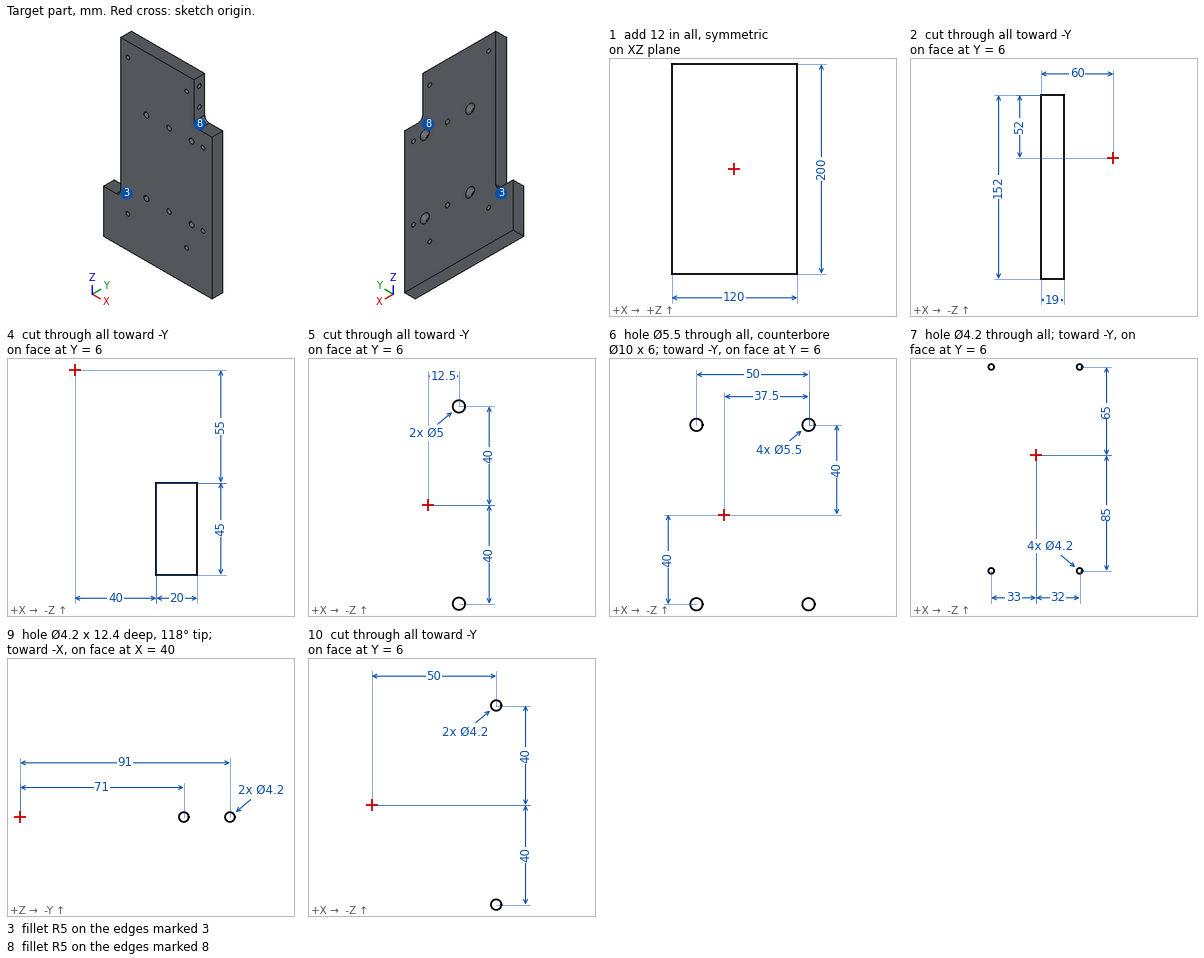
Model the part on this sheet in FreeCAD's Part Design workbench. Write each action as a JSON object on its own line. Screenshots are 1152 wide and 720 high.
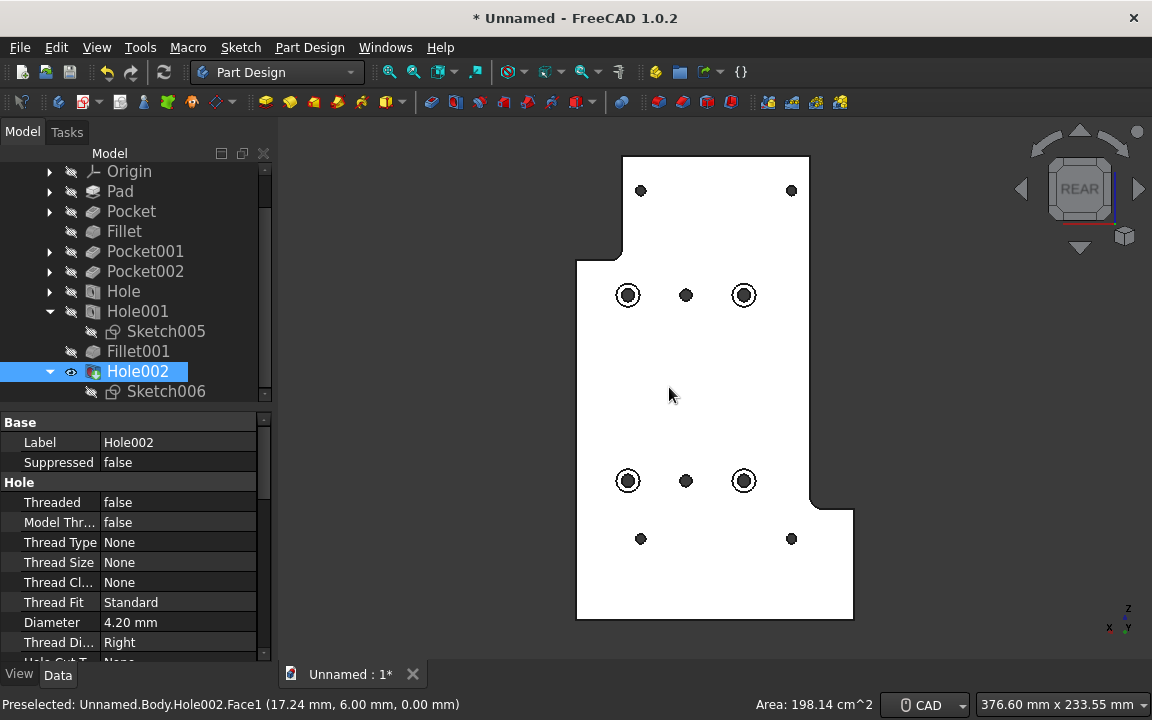
{"action": "left_click", "coordinate": [84, 102]}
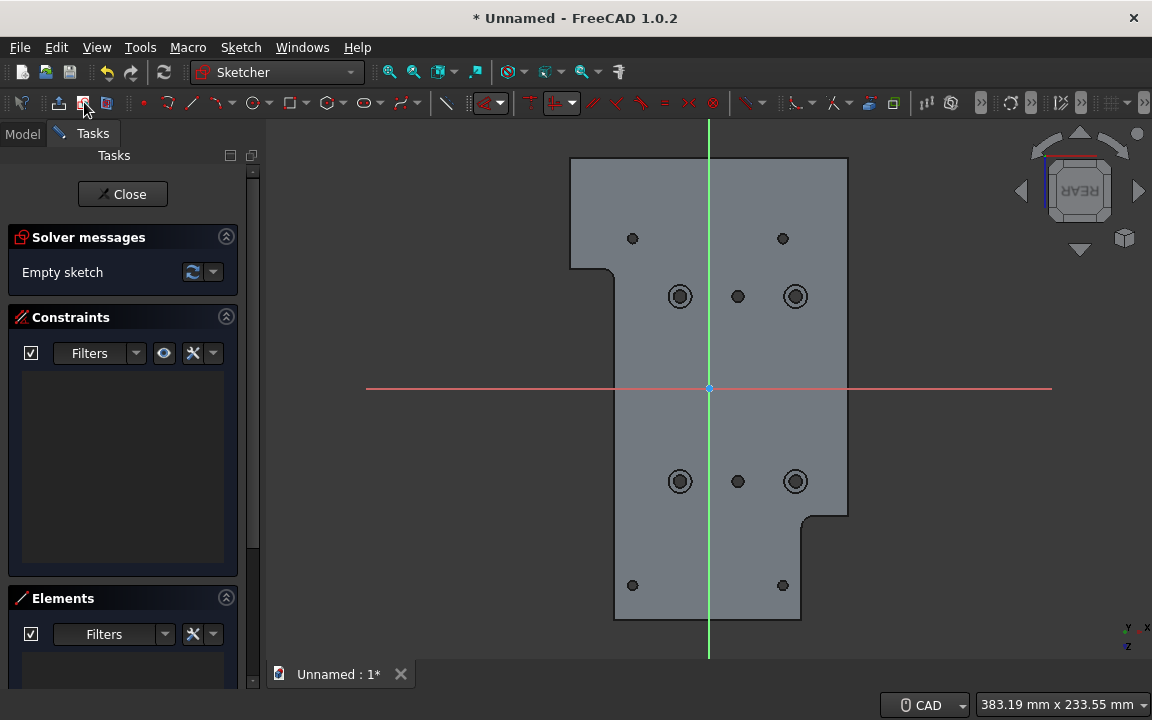
{"action": "scroll", "coordinate": [926, 389], "scroll_direction": "up", "scroll_amount": 3}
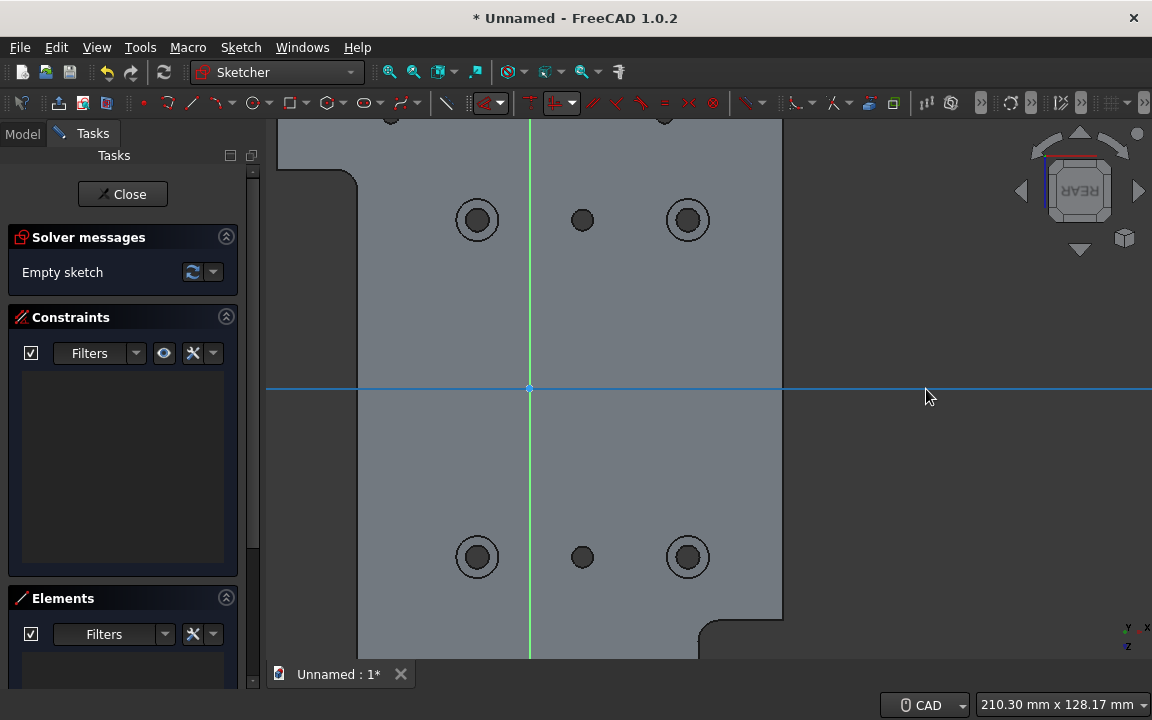
{"action": "left_click", "coordinate": [254, 104]}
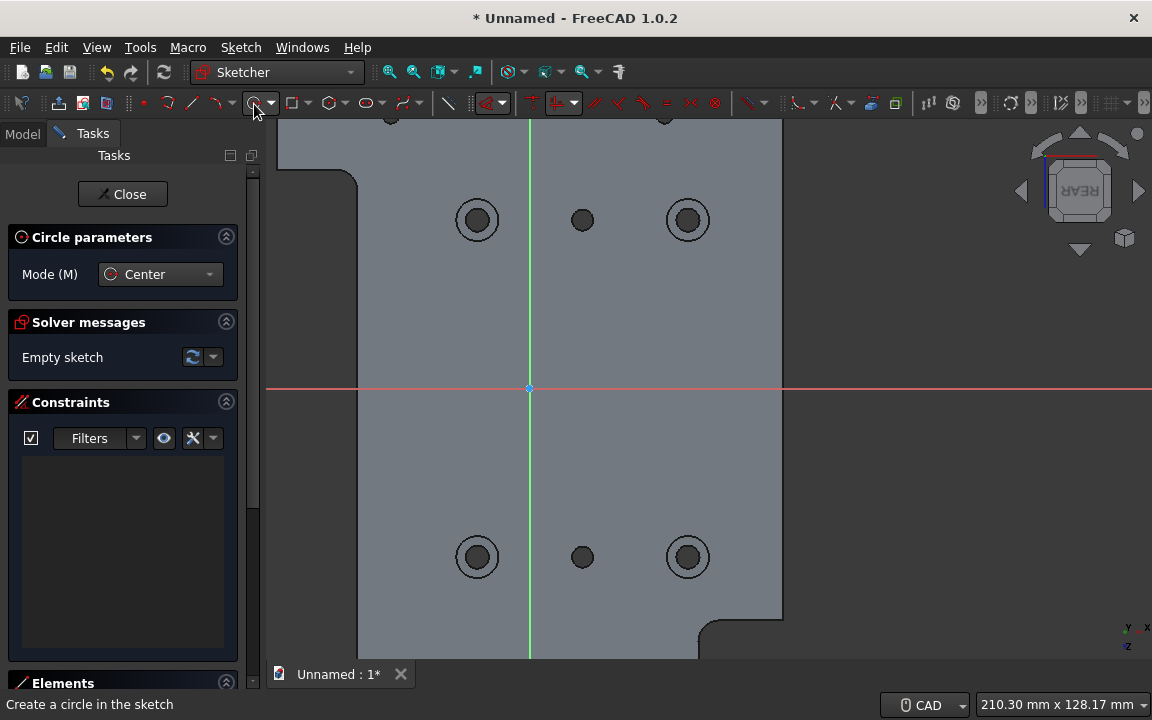
{"action": "scroll", "coordinate": [741, 220], "scroll_direction": "up", "scroll_amount": 5}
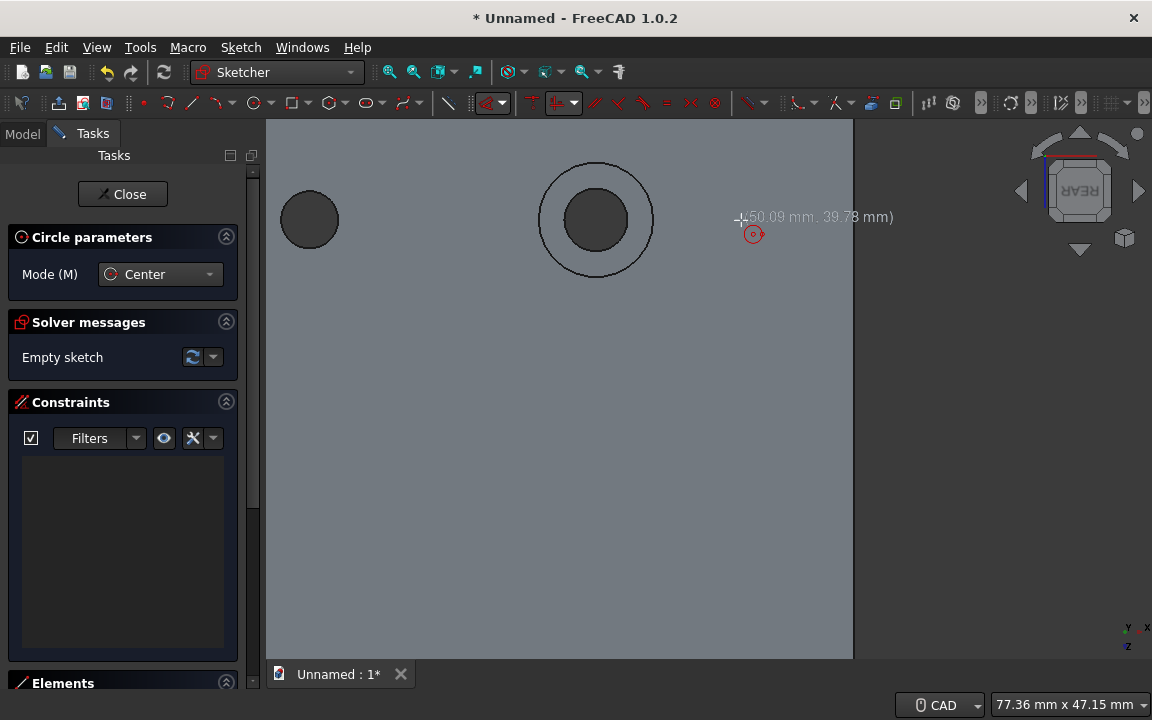
{"action": "left_click", "coordinate": [739, 220]}
{"action": "left_click", "coordinate": [756, 203]}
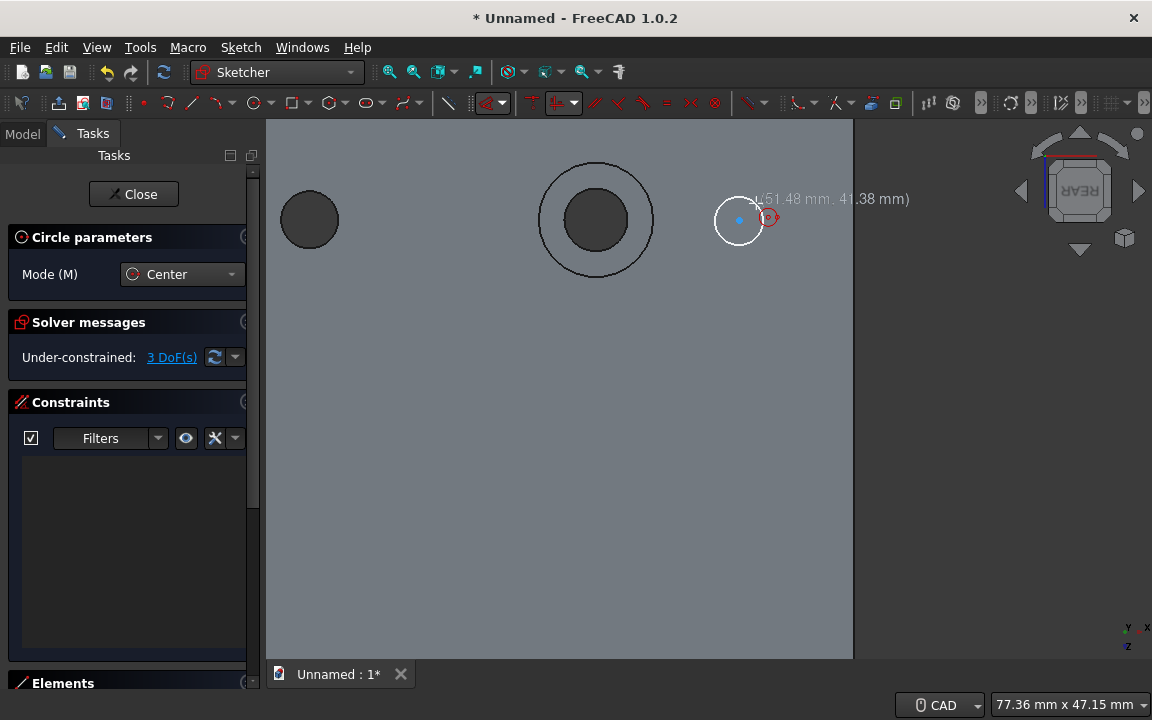
{"action": "scroll", "coordinate": [743, 221], "scroll_direction": "down", "scroll_amount": 5}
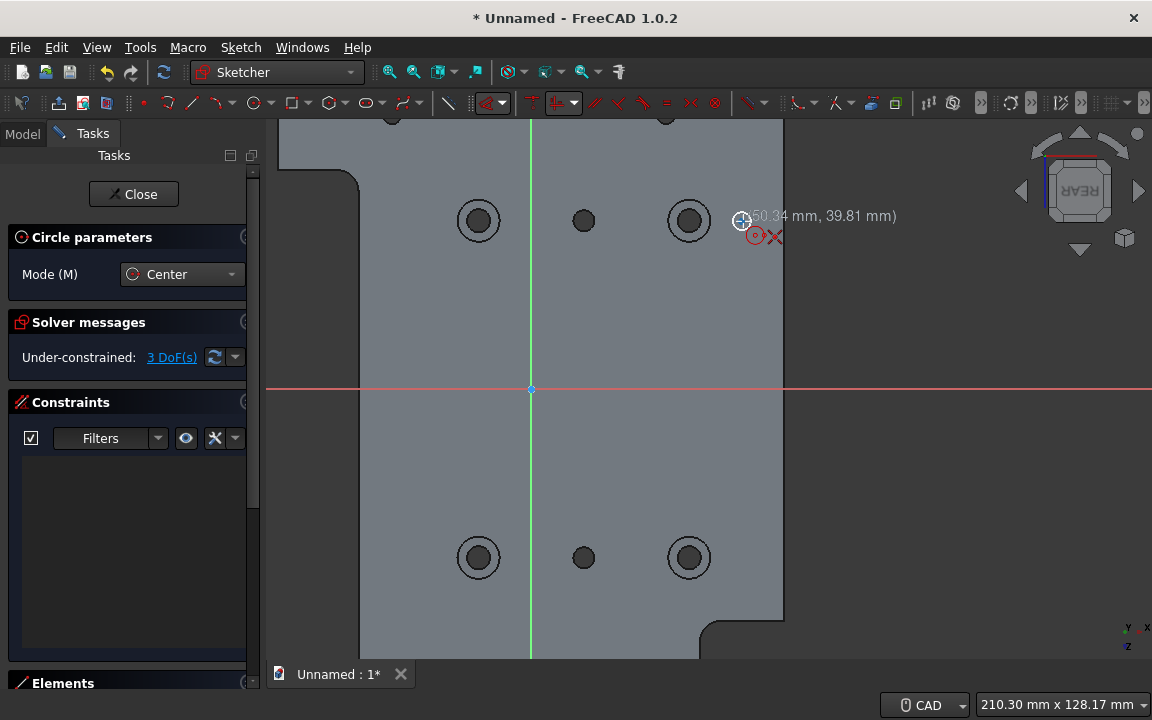
{"action": "scroll", "coordinate": [742, 558], "scroll_direction": "up", "scroll_amount": 5}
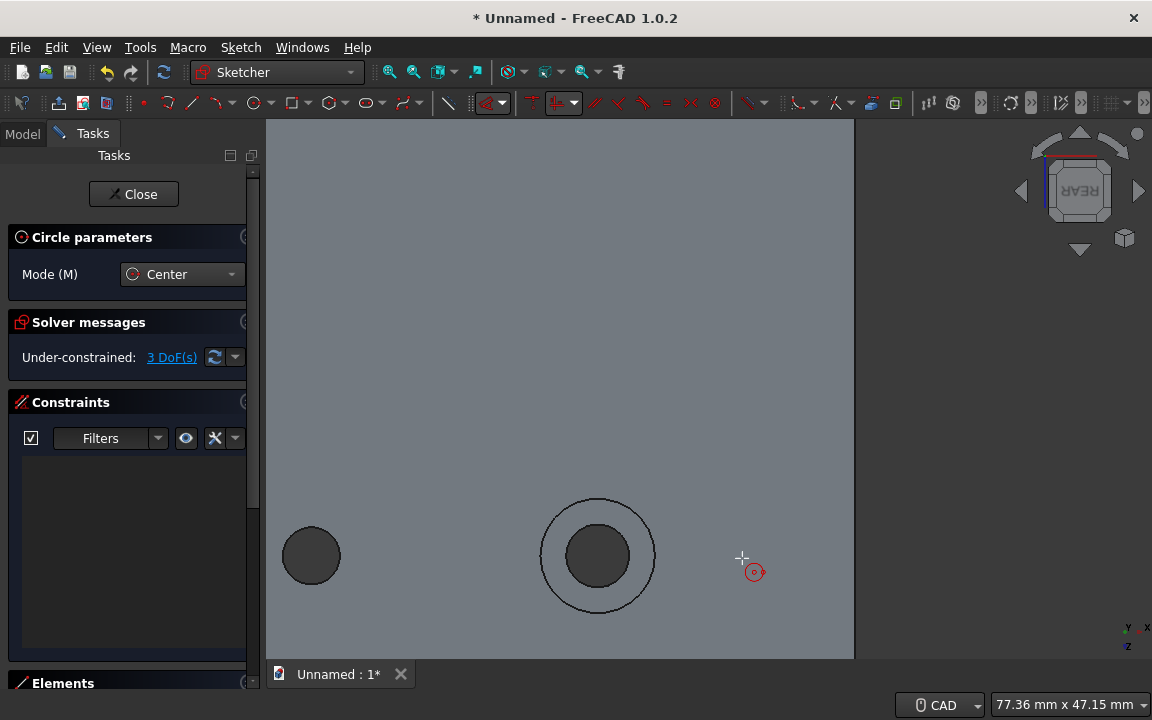
{"action": "left_click", "coordinate": [741, 556]}
{"action": "left_click", "coordinate": [758, 539]}
{"action": "key", "text": "Escape"}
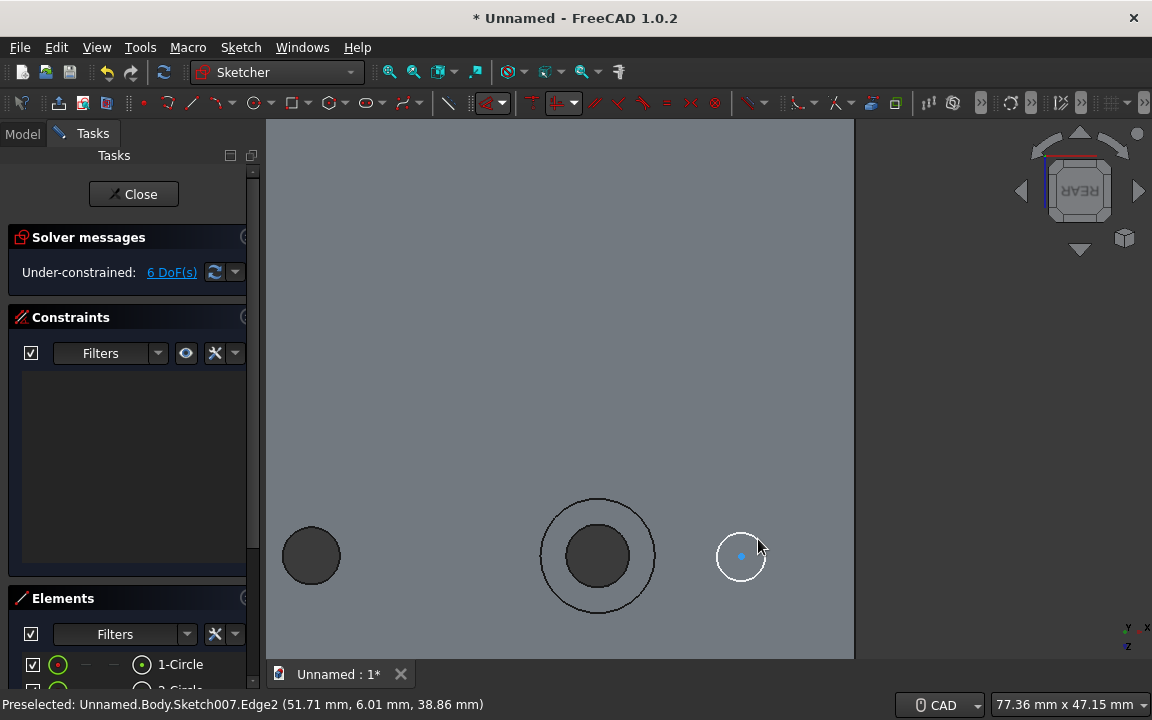
{"action": "scroll", "coordinate": [742, 558], "scroll_direction": "down", "scroll_amount": 5}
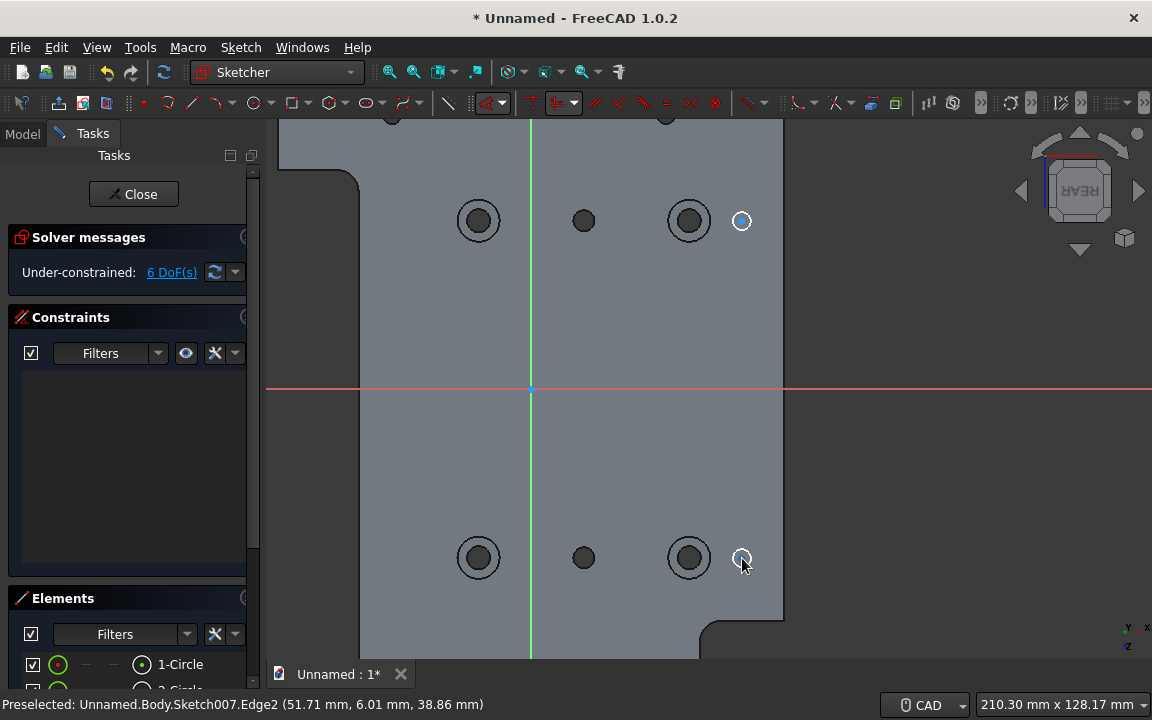
{"action": "scroll", "coordinate": [748, 215], "scroll_direction": "up", "scroll_amount": 3}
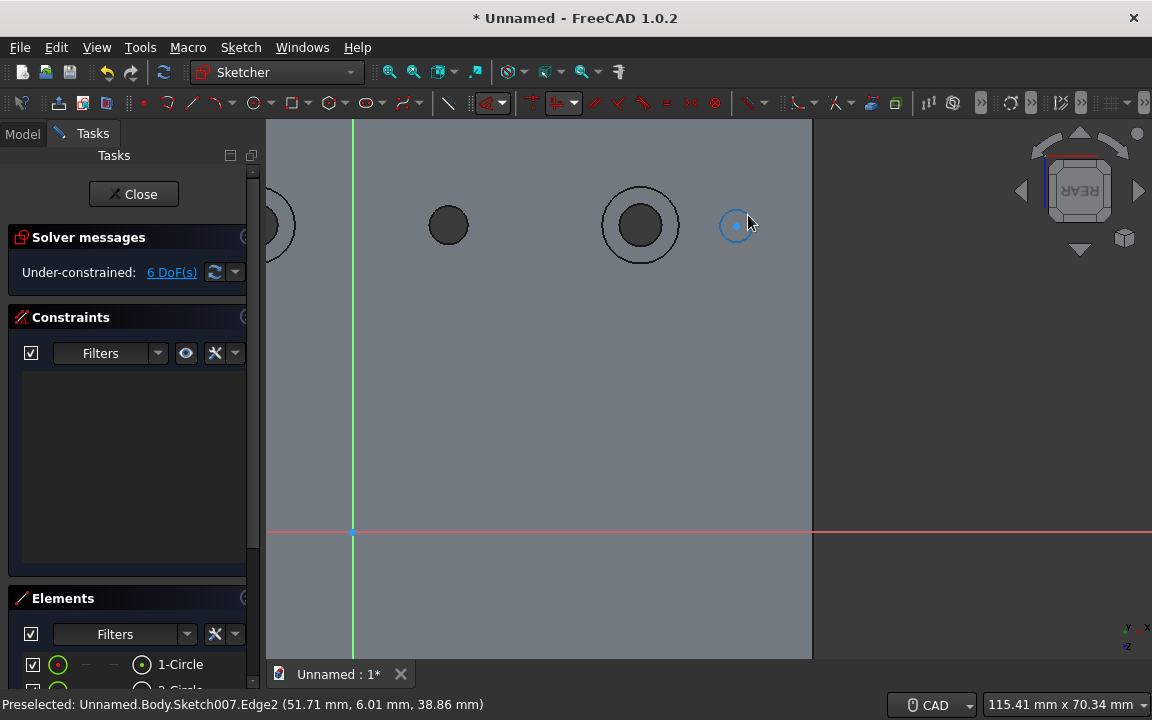
{"action": "left_click", "coordinate": [748, 215]}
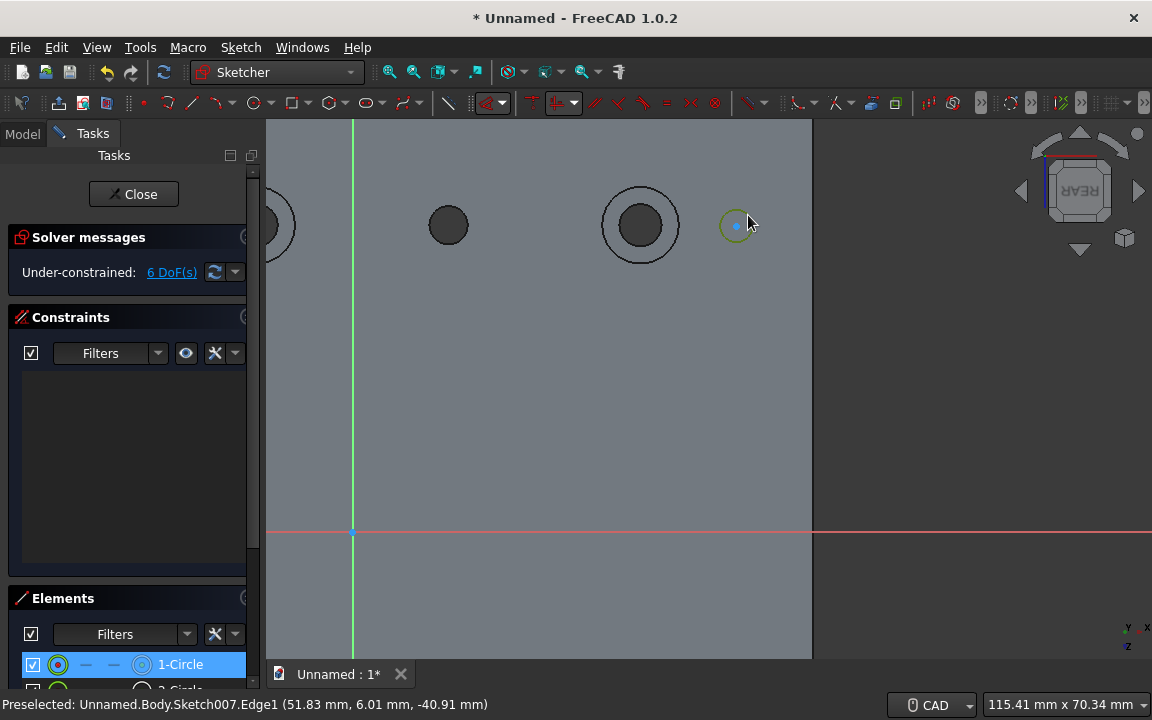
{"action": "scroll", "coordinate": [747, 215], "scroll_direction": "down", "scroll_amount": 3}